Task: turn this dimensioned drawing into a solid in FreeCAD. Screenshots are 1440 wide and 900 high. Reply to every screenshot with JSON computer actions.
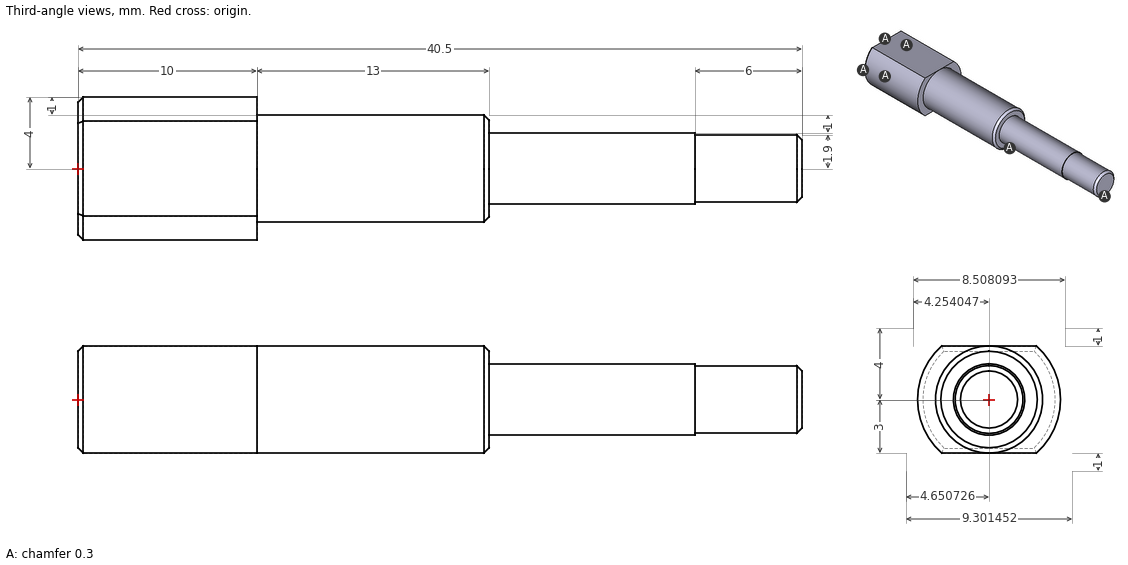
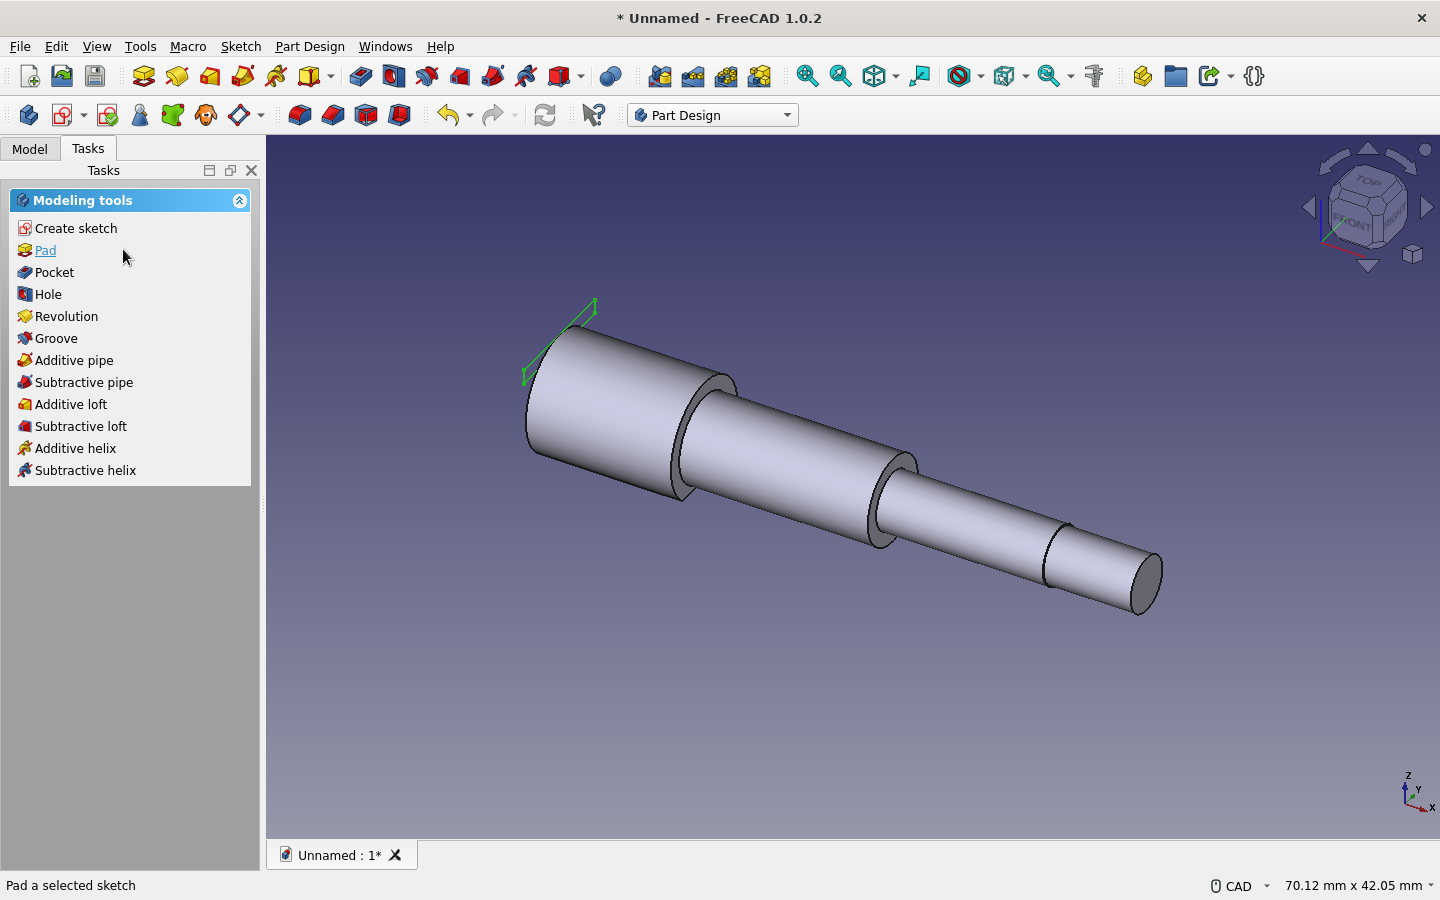
{"action": "left_click", "coordinate": [361, 76]}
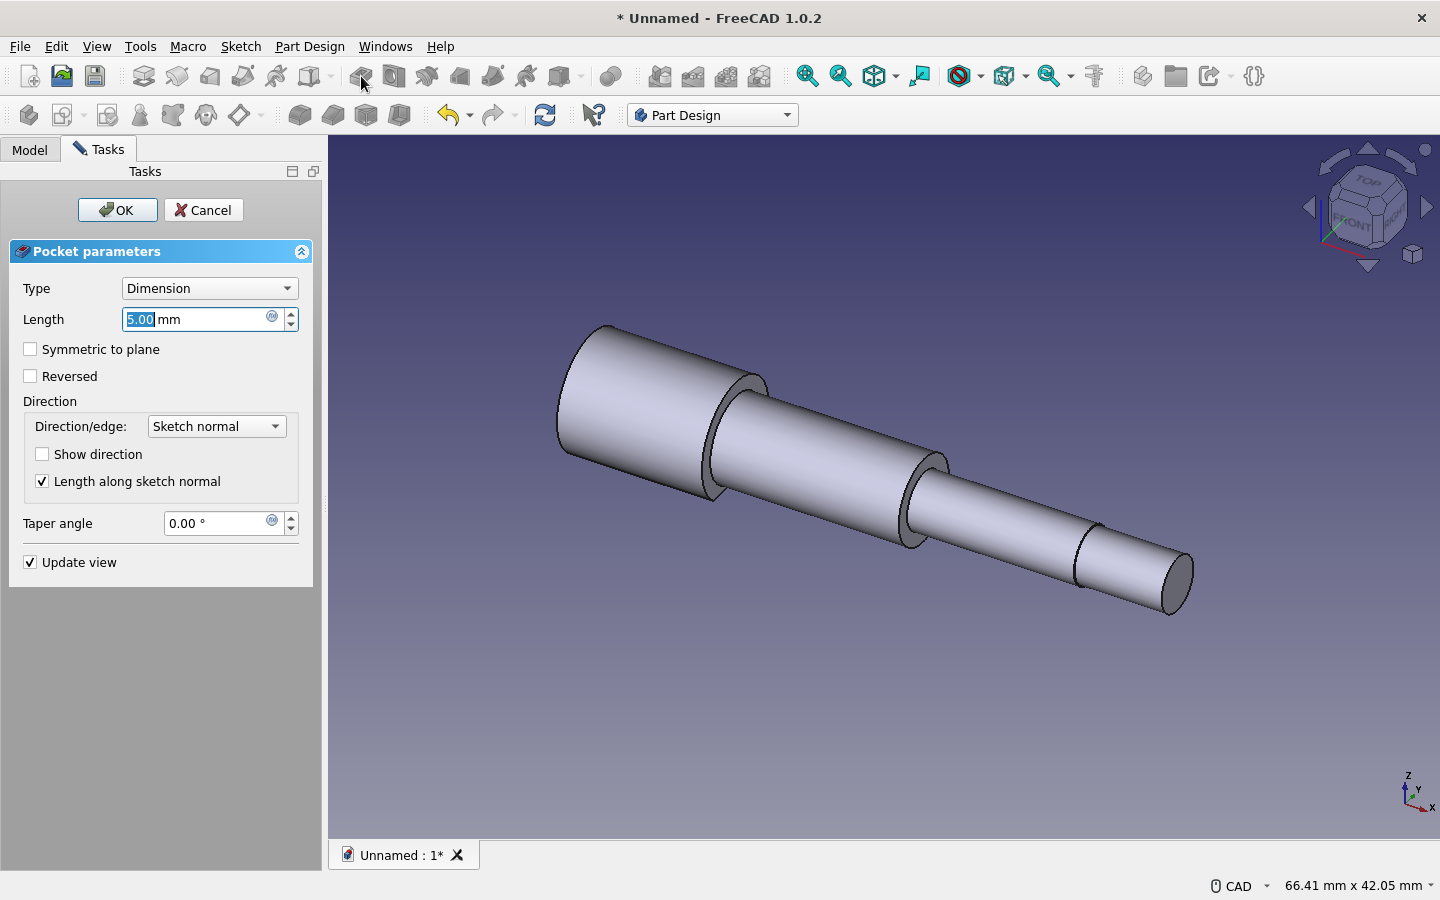
{"action": "left_click", "coordinate": [210, 288]}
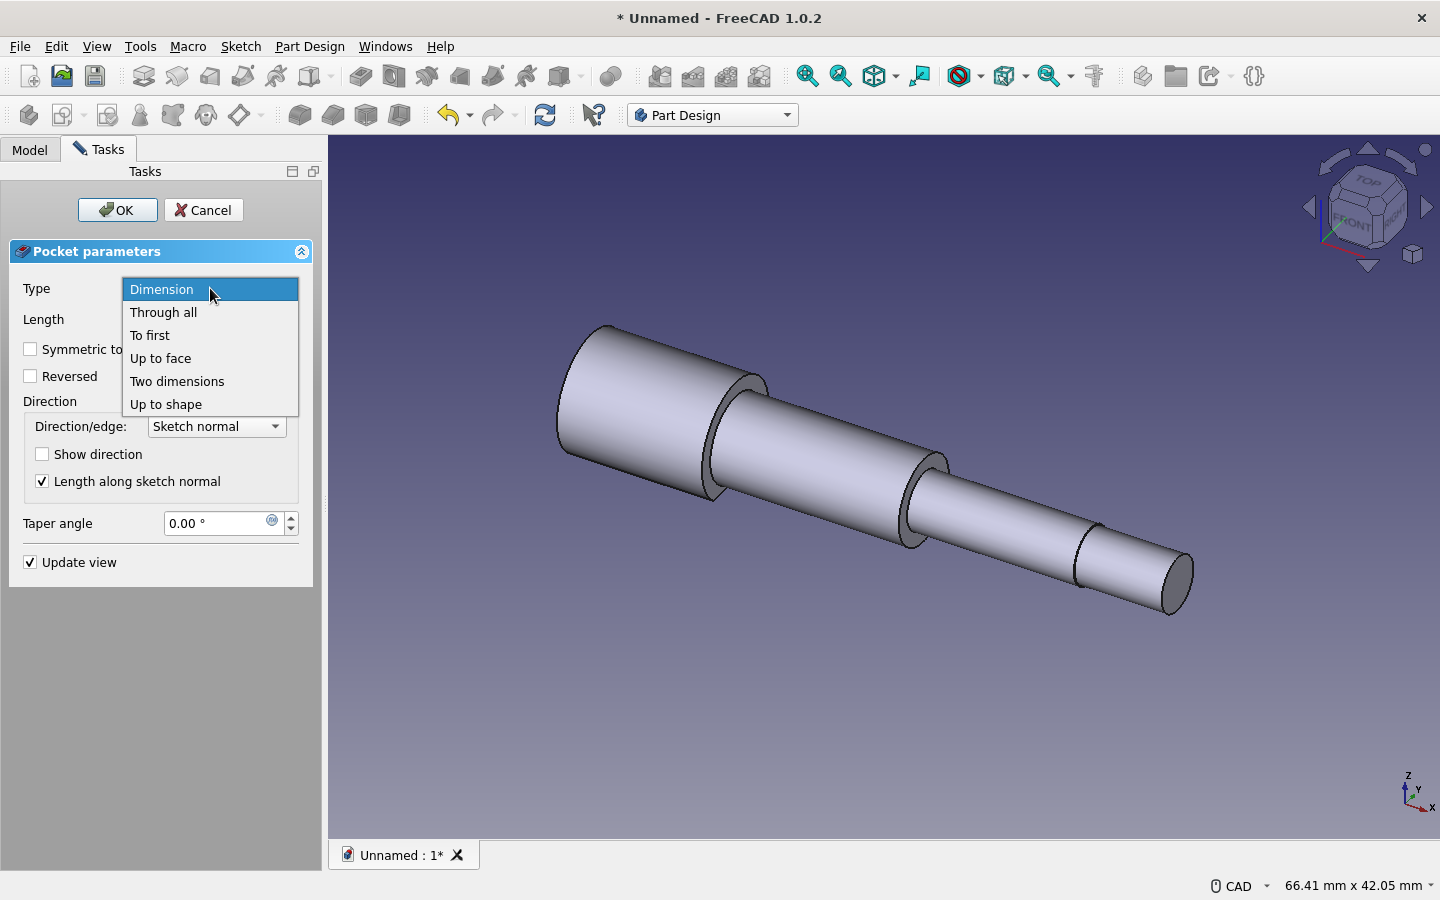
{"action": "left_click", "coordinate": [208, 336]}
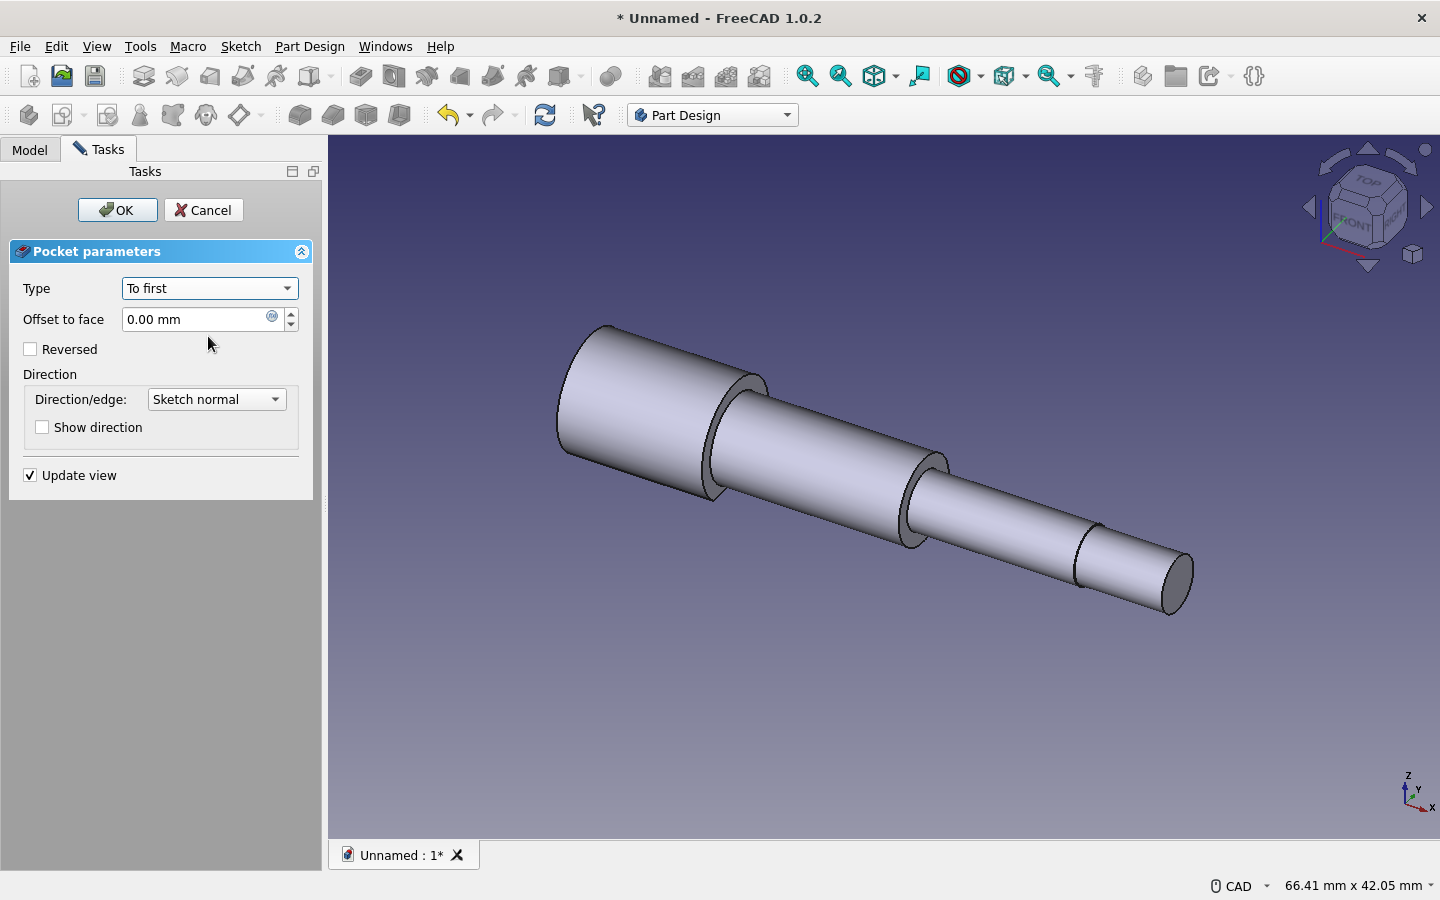
{"action": "left_click", "coordinate": [31, 349]}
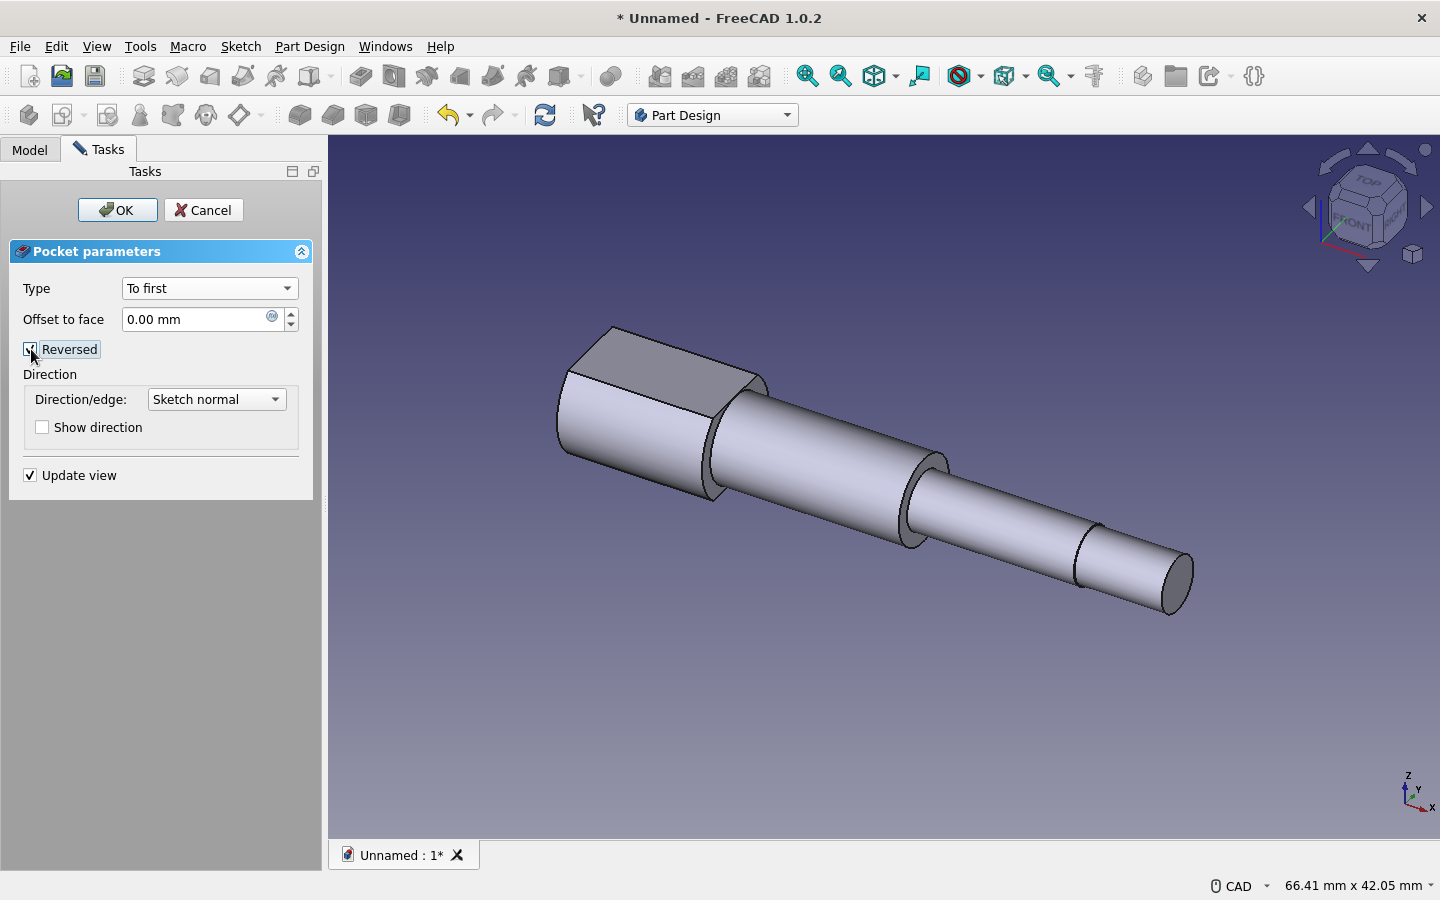
{"action": "left_click", "coordinate": [118, 210]}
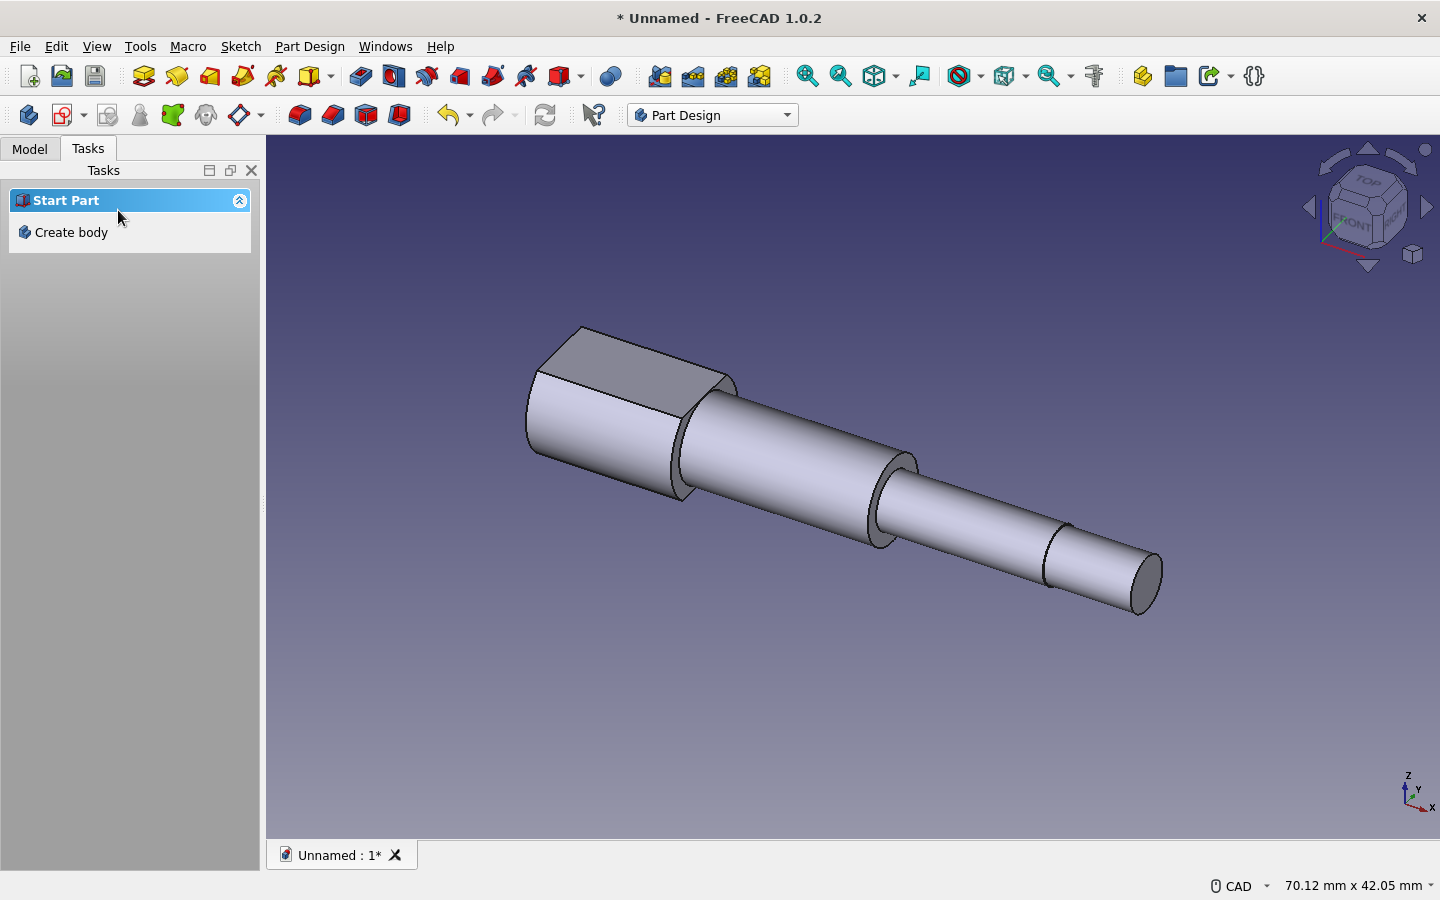
{"action": "left_click", "coordinate": [868, 524]}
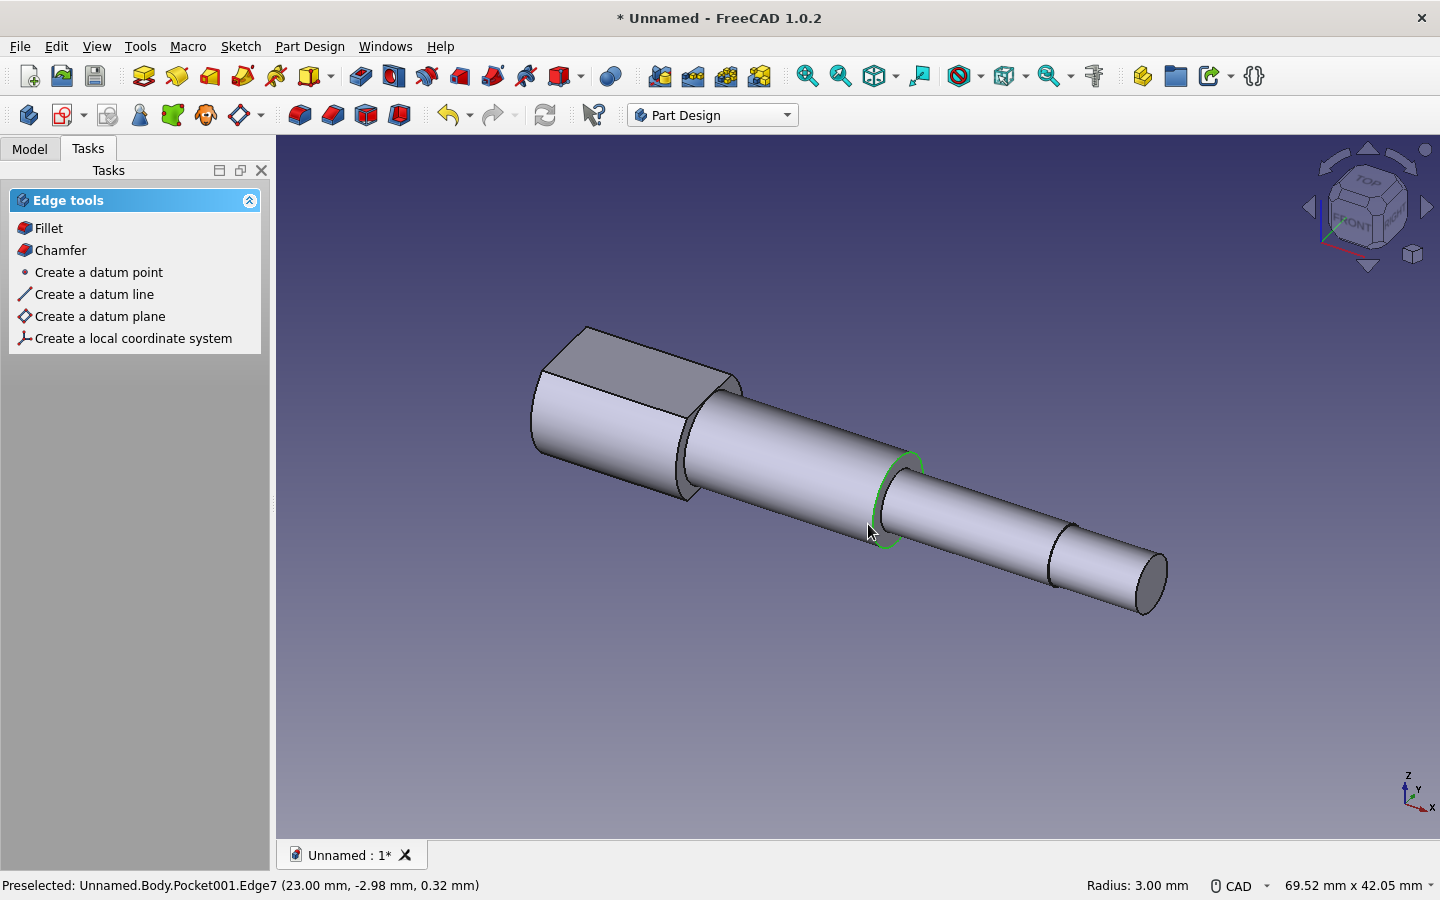
{"action": "left_click", "coordinate": [1136, 599], "text": "ctrl"}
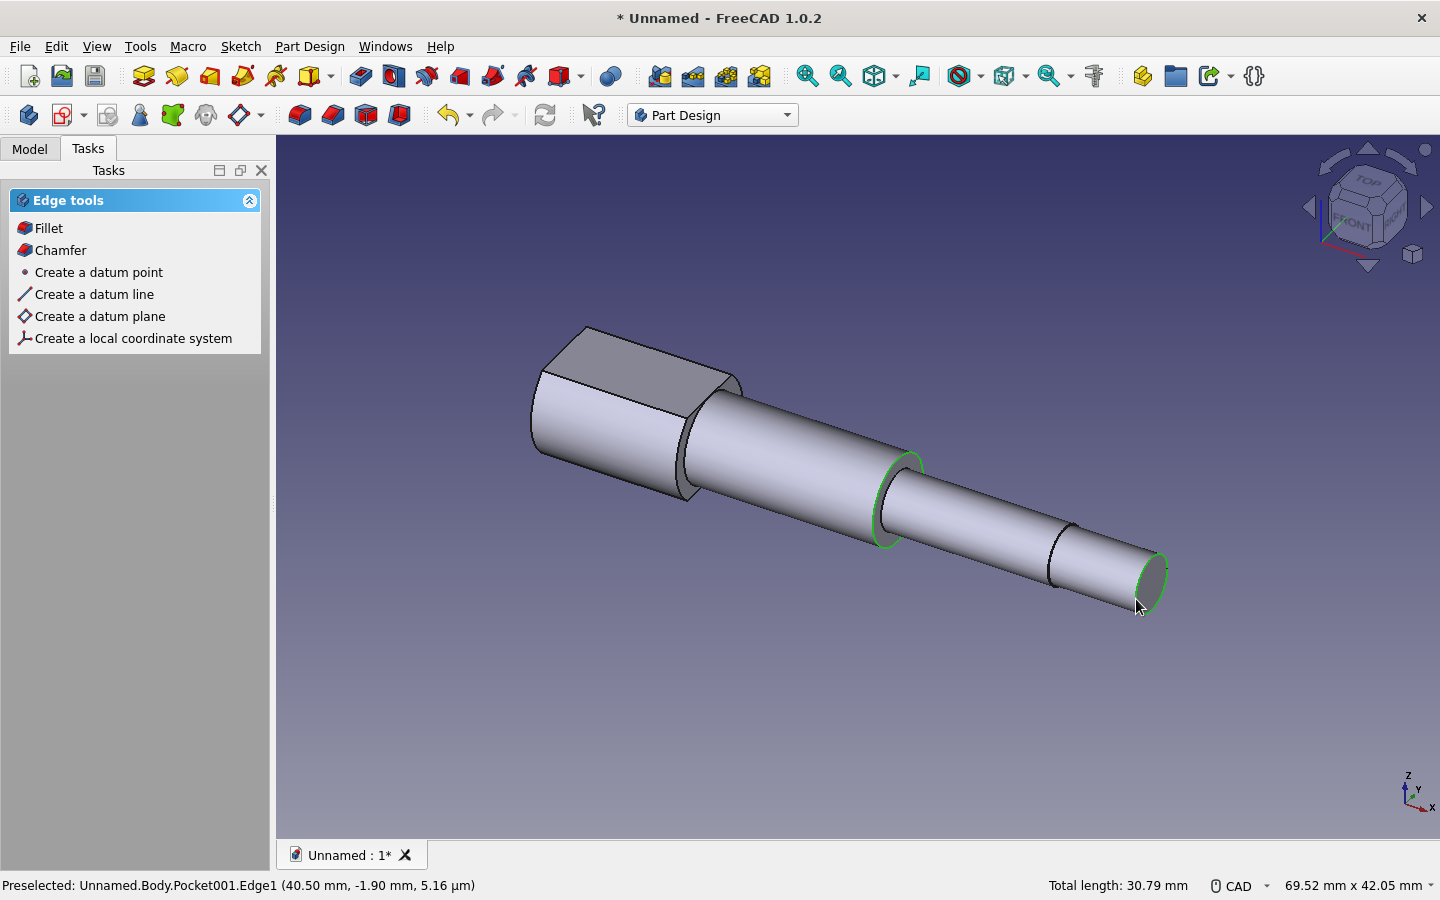
{"action": "key", "text": "0"}